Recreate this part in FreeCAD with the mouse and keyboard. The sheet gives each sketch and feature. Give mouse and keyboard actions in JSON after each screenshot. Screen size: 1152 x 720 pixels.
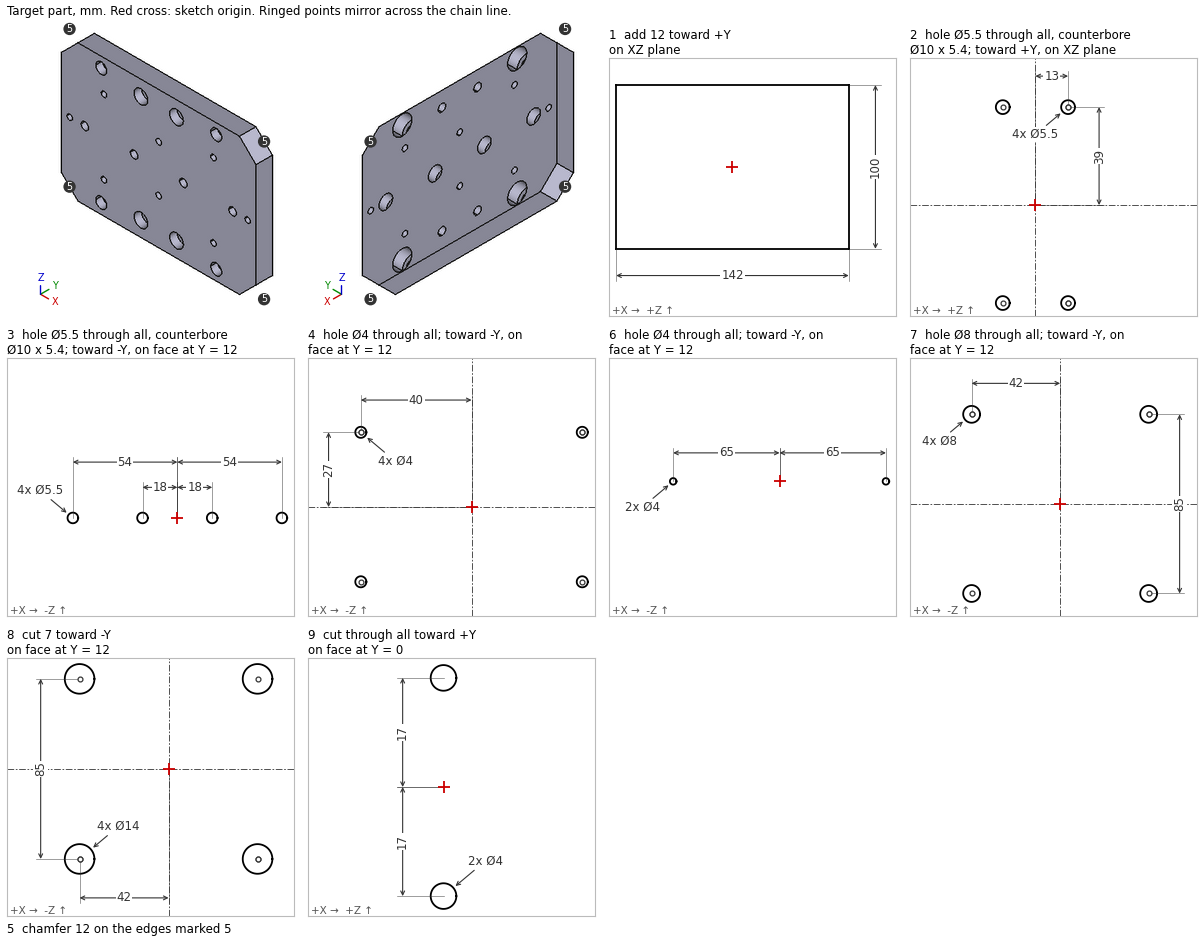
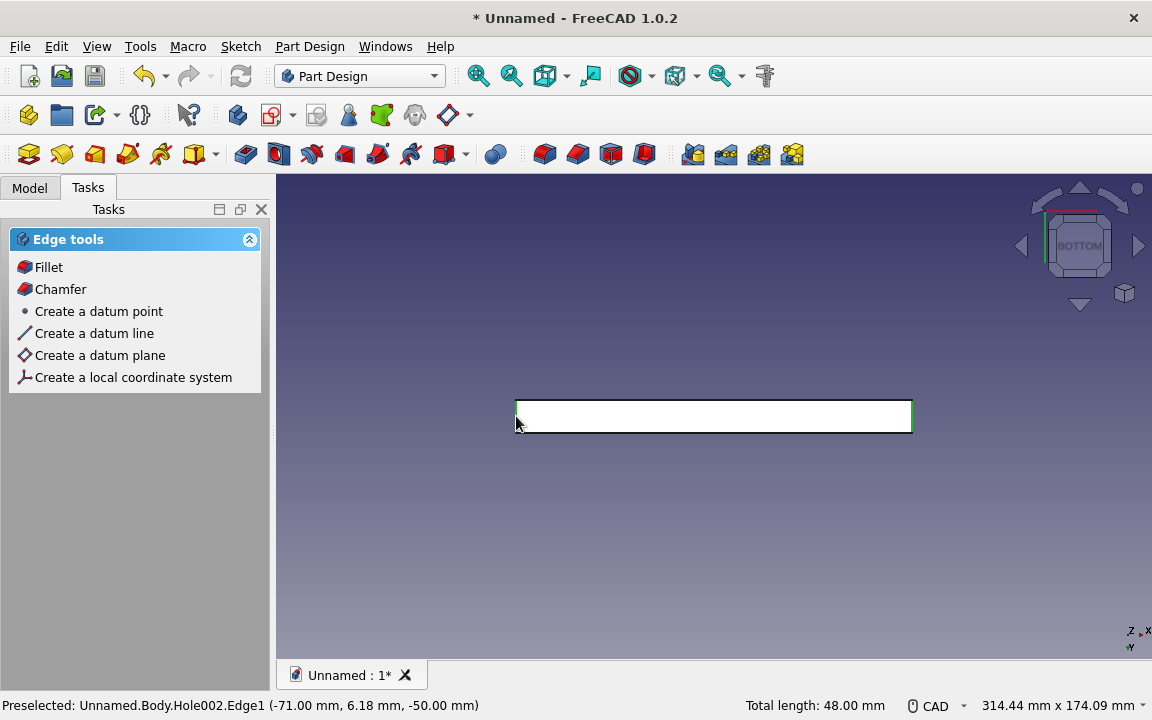
{"action": "left_click", "coordinate": [578, 154]}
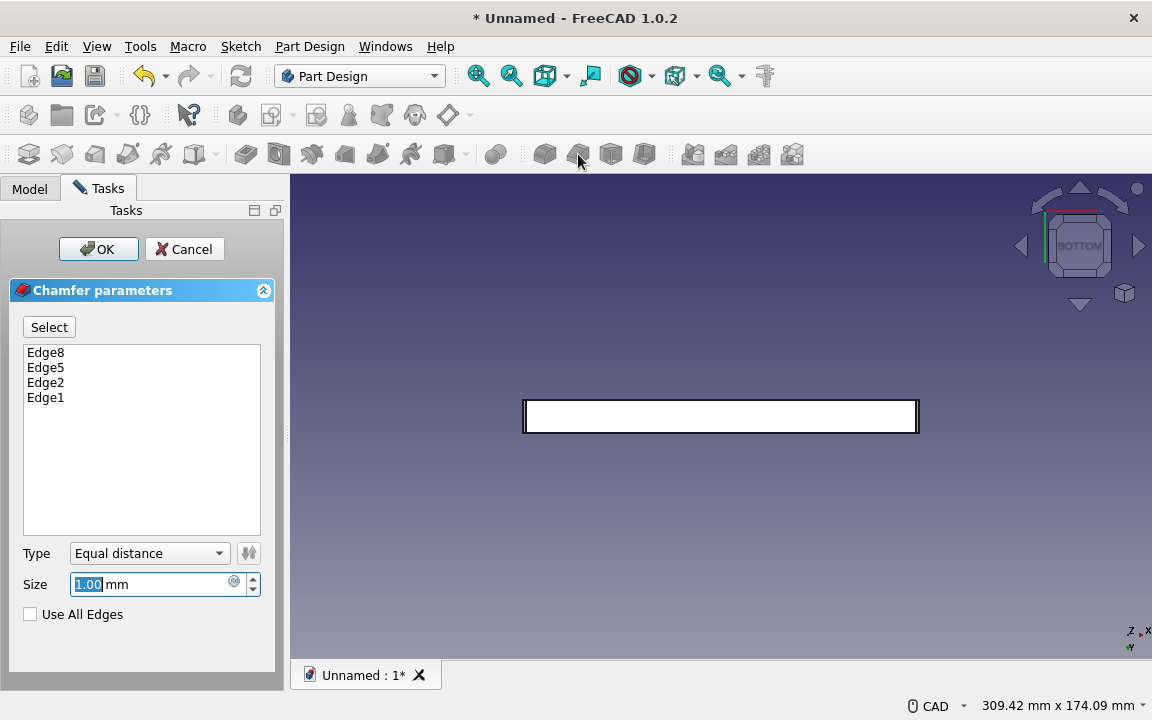
{"action": "type", "text": "12"}
{"action": "key", "text": "Tab"}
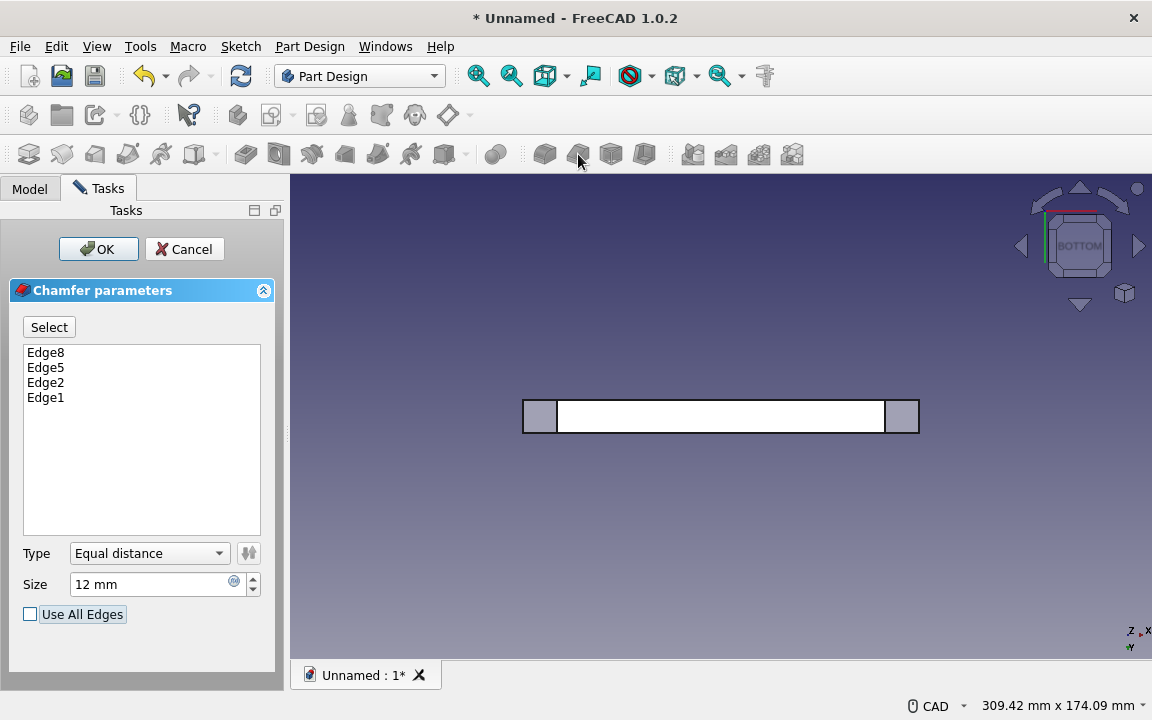
{"action": "left_click", "coordinate": [99, 249]}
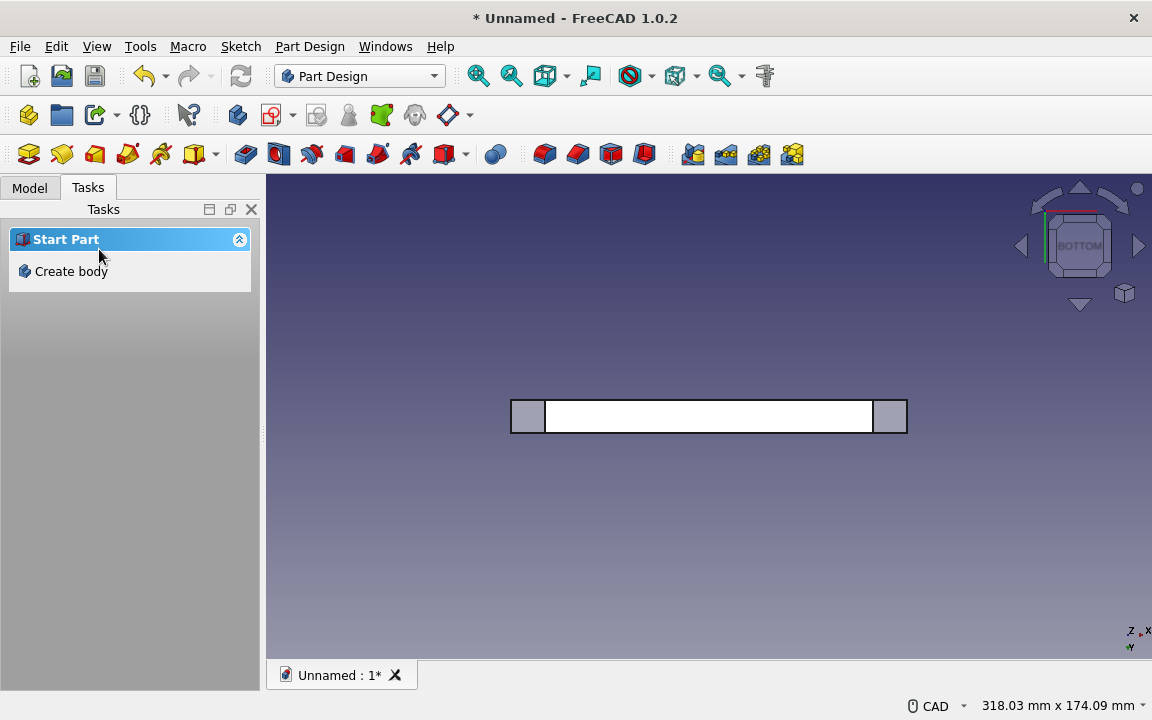
{"action": "left_click", "coordinate": [479, 76]}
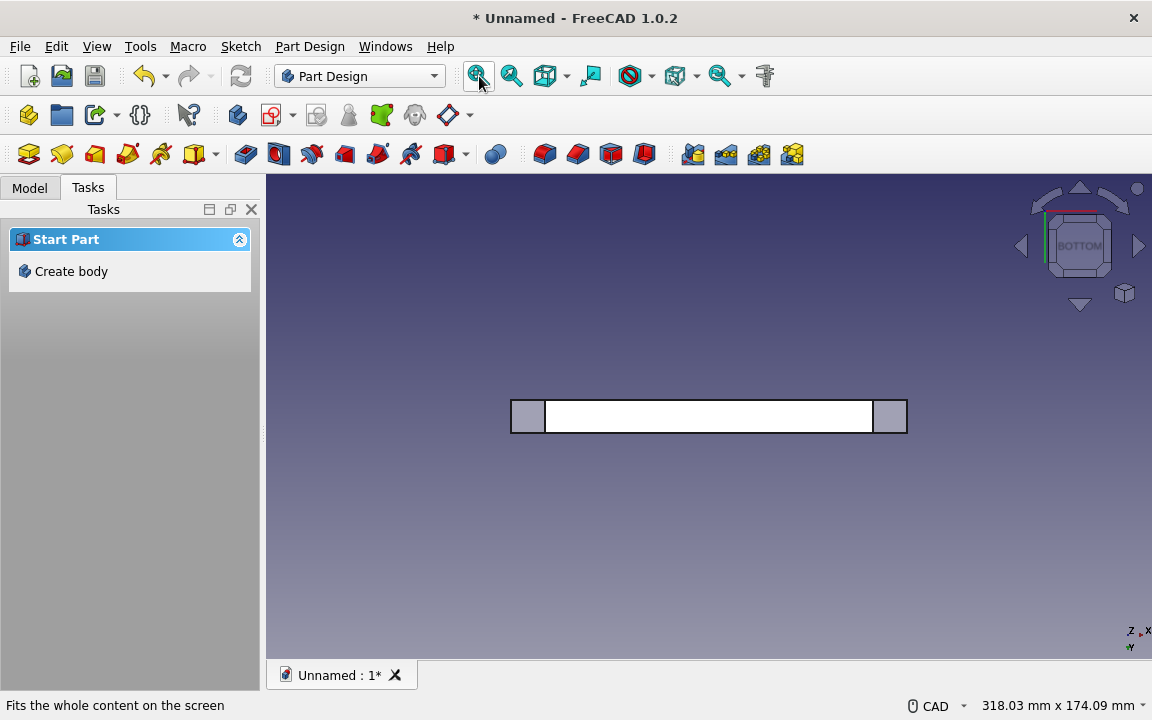
{"action": "key", "text": "4"}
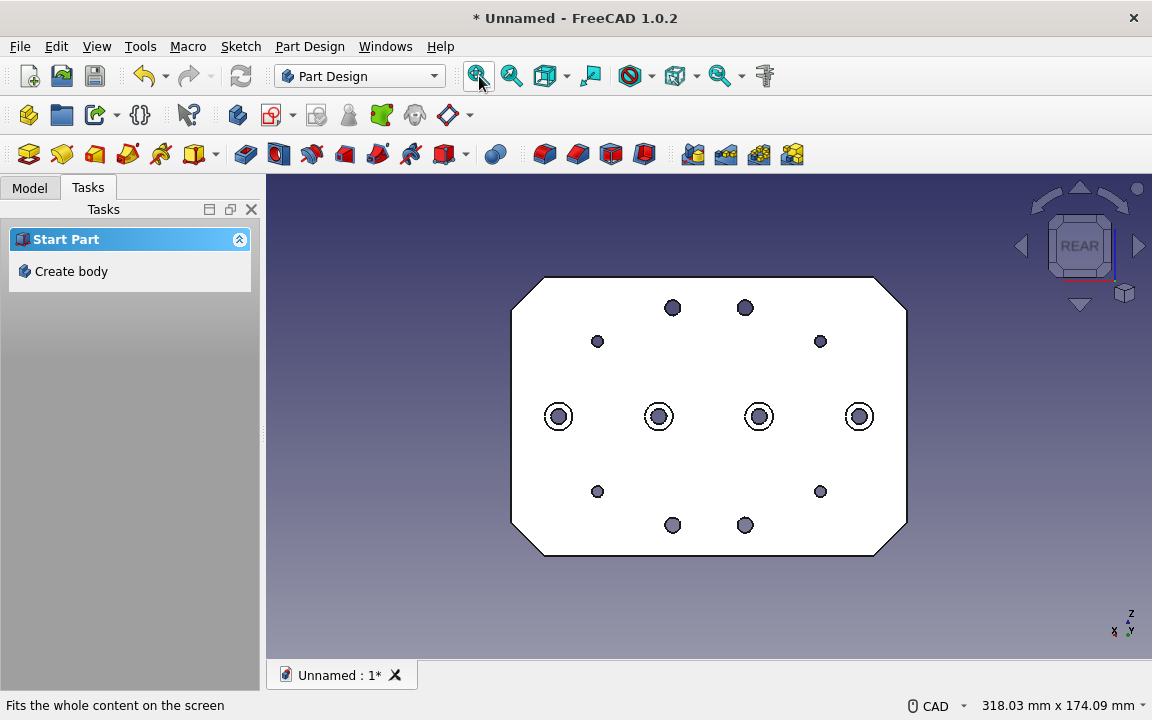
{"action": "left_click", "coordinate": [709, 455]}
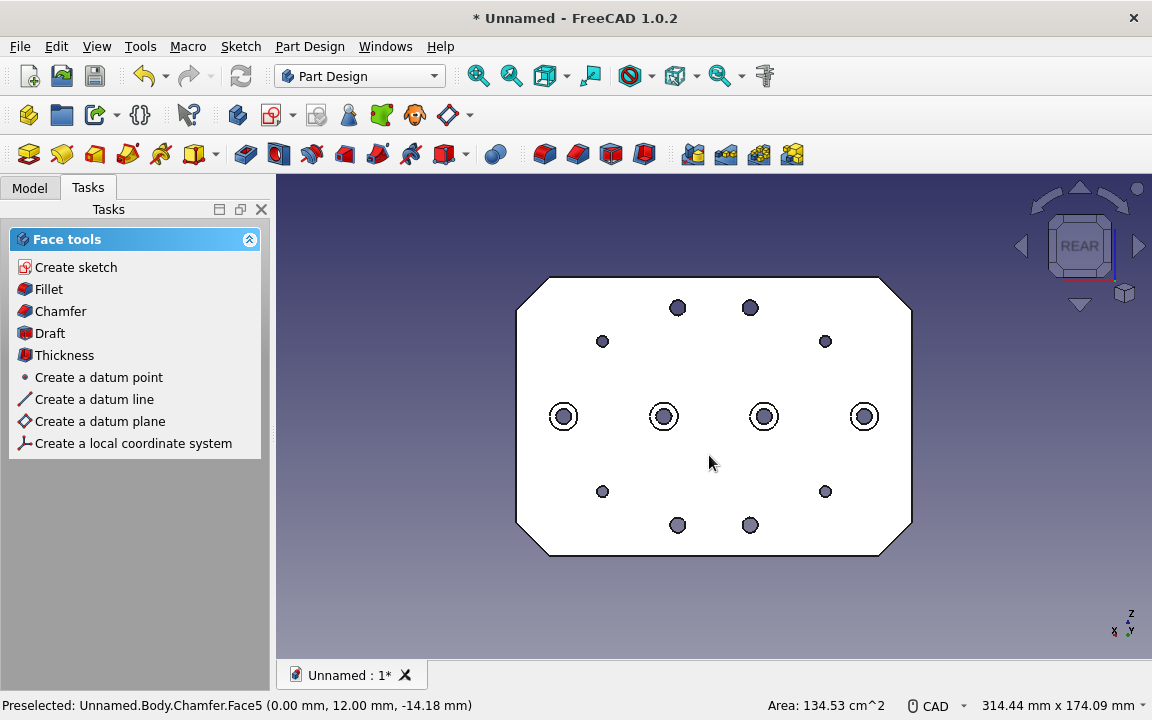
{"action": "left_click", "coordinate": [270, 116]}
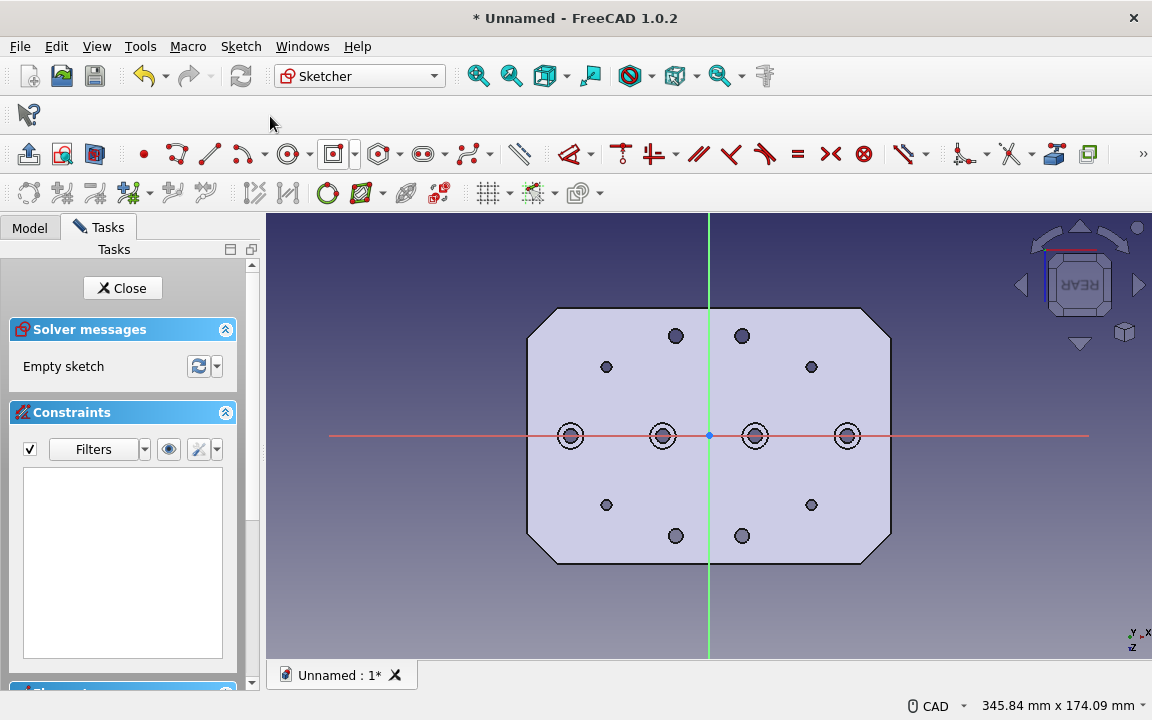
{"action": "scroll", "coordinate": [848, 436], "scroll_direction": "up", "scroll_amount": 2}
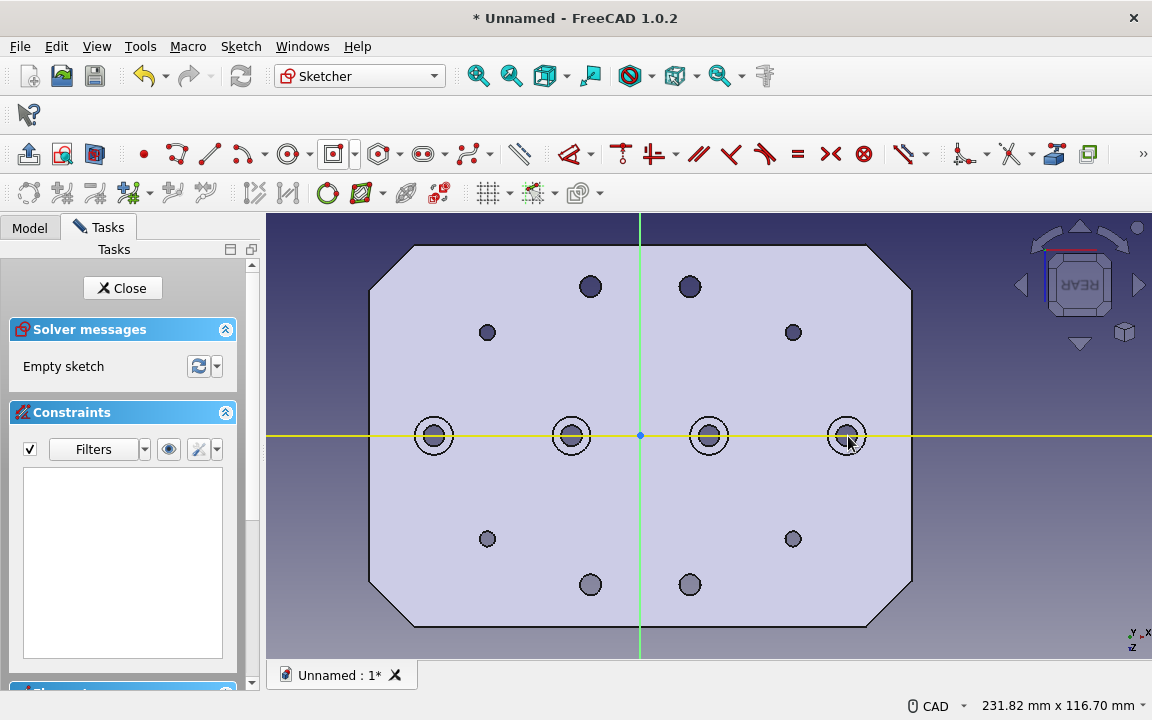
{"action": "left_click", "coordinate": [288, 154]}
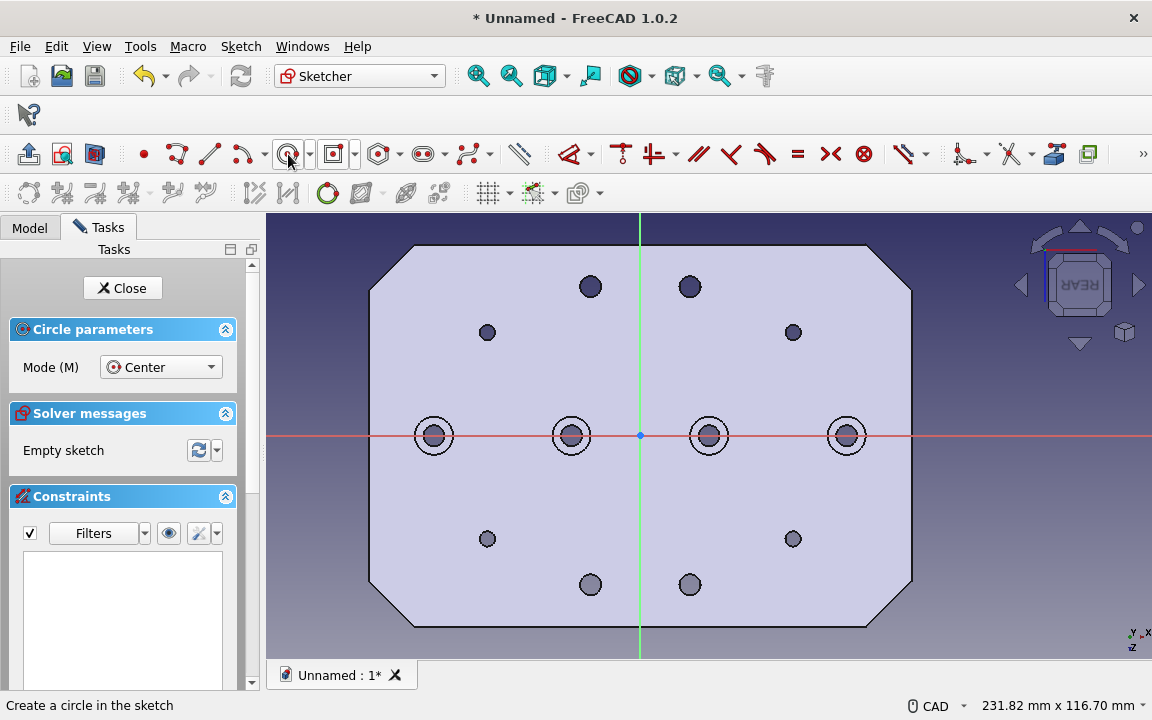
{"action": "scroll", "coordinate": [392, 436], "scroll_direction": "up", "scroll_amount": 6}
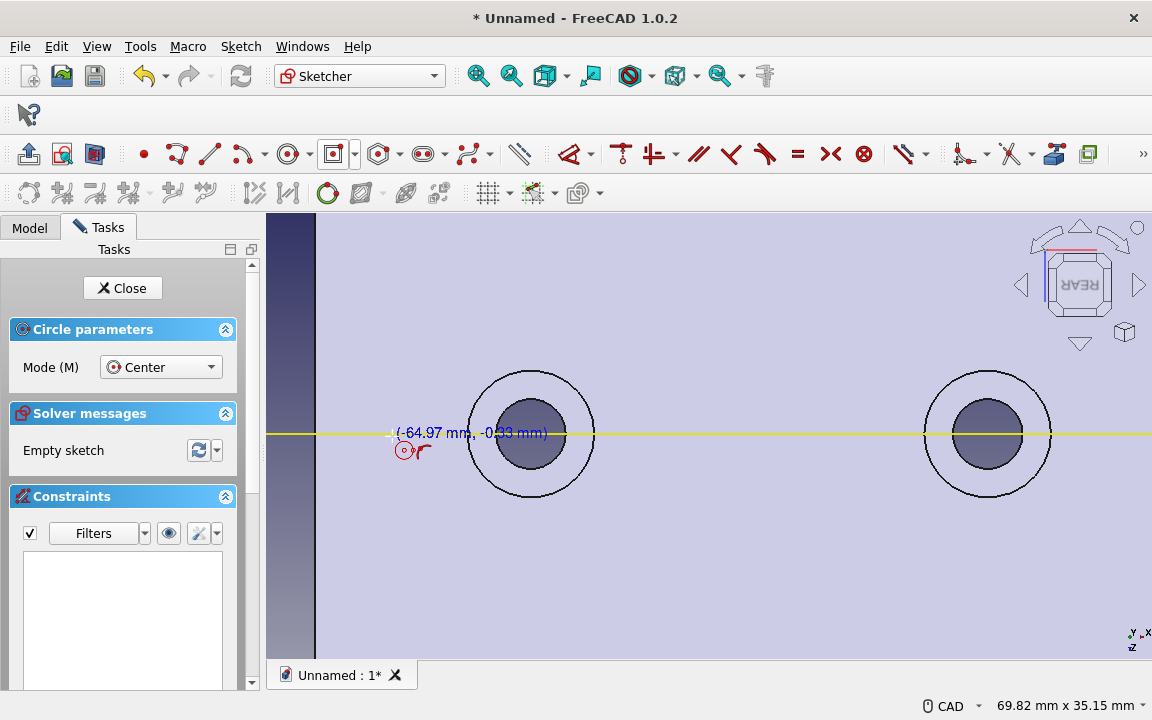
{"action": "left_click", "coordinate": [391, 434]}
{"action": "left_click", "coordinate": [409, 416]}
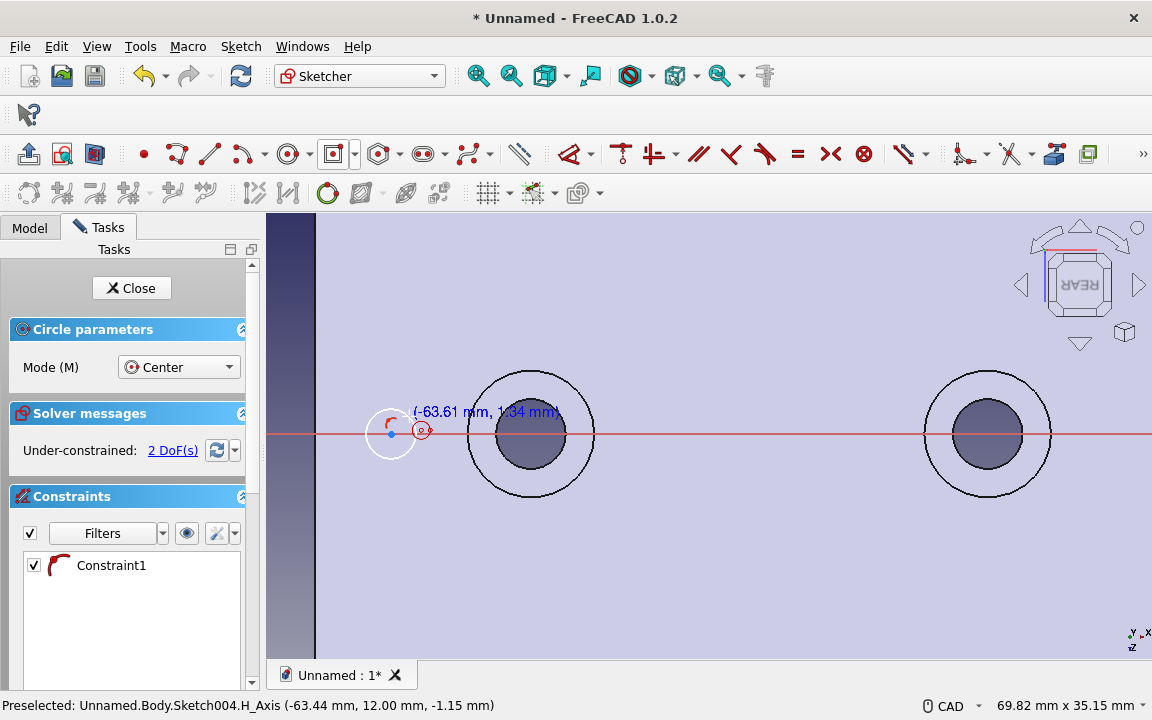
{"action": "scroll", "coordinate": [392, 437], "scroll_direction": "down", "scroll_amount": 6}